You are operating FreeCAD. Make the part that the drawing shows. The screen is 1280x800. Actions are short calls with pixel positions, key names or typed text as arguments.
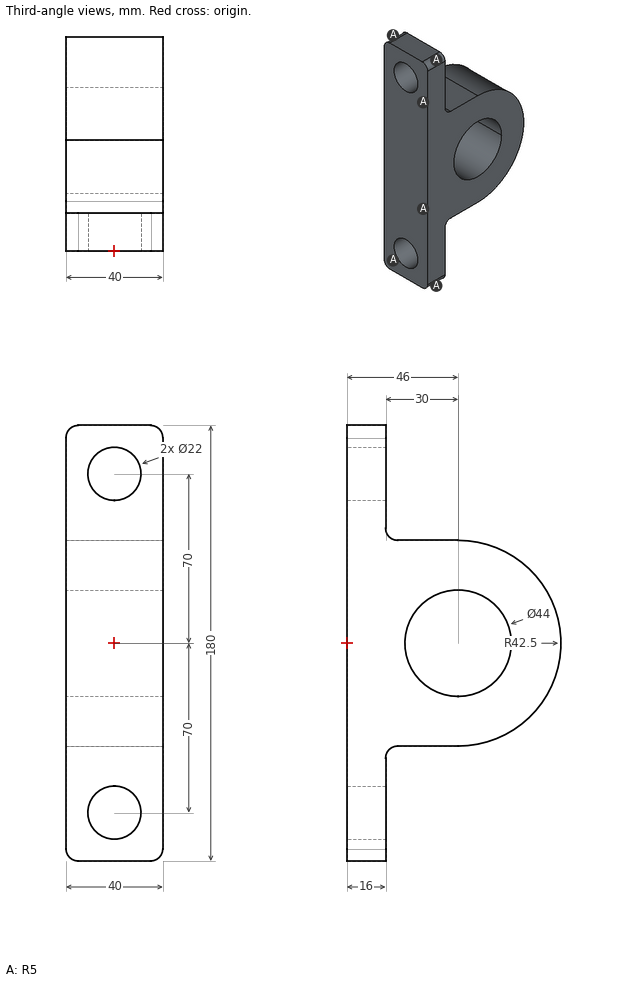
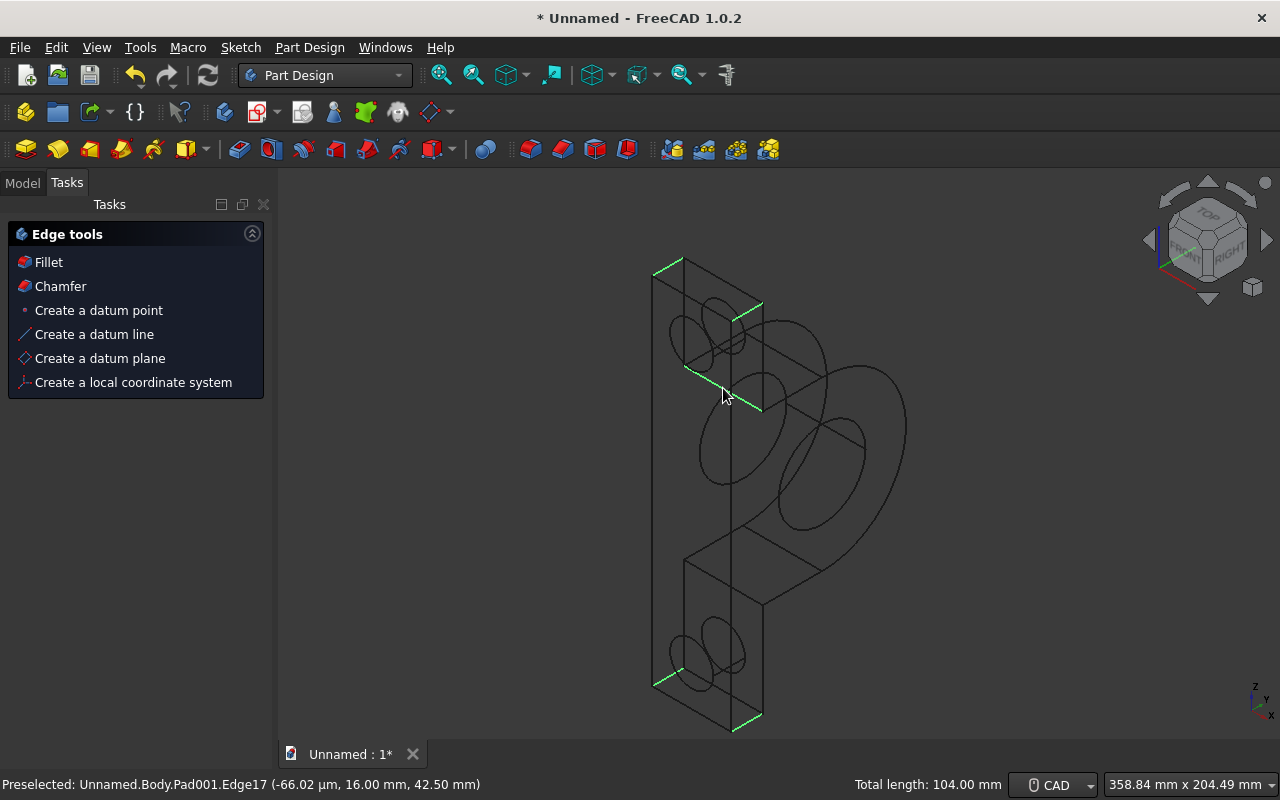
click(723, 582, ctrl)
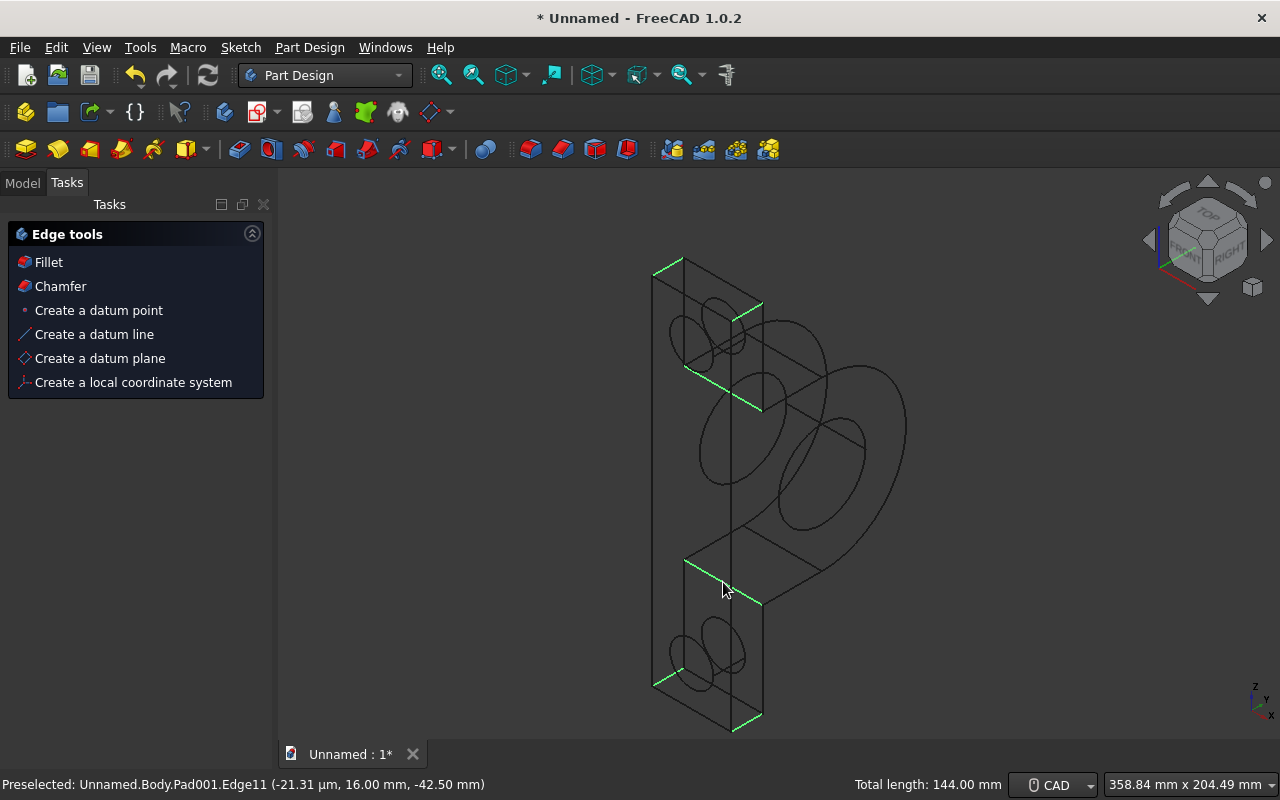
key(v)
key(1)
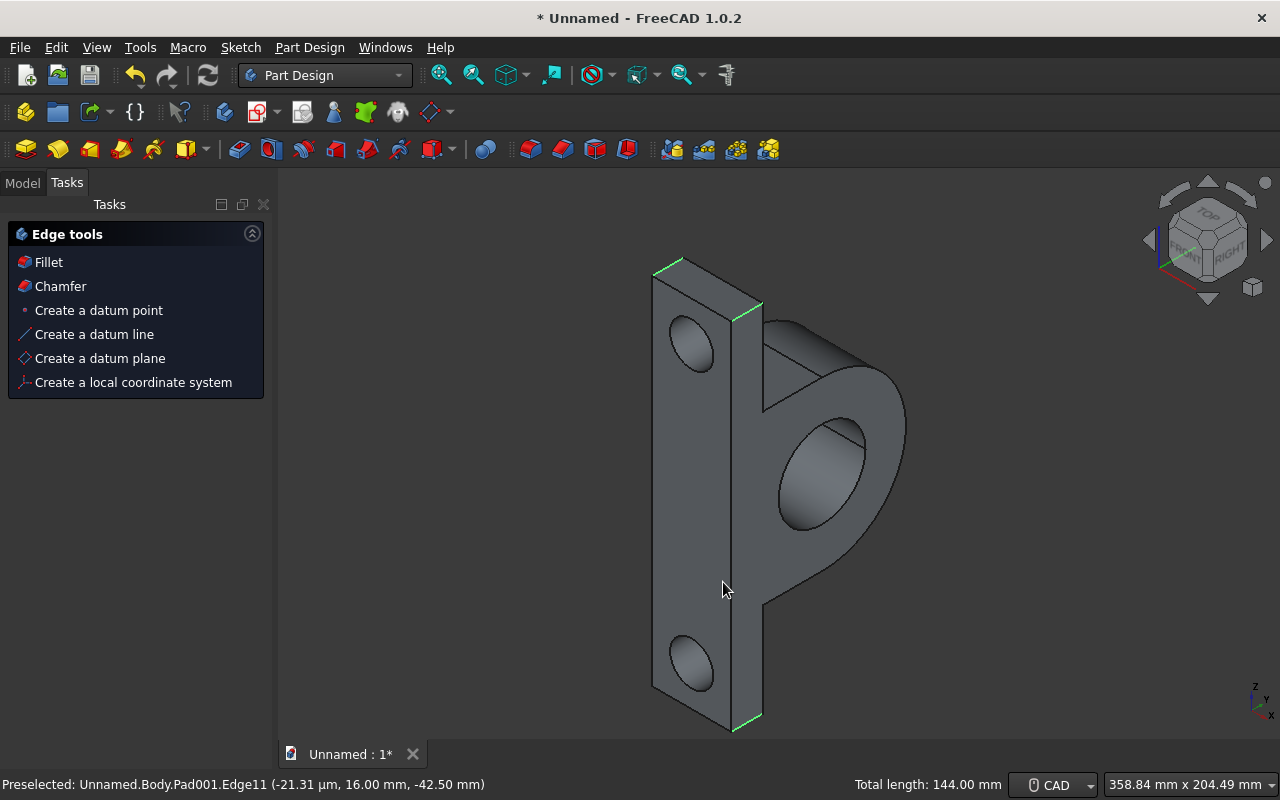
click(532, 150)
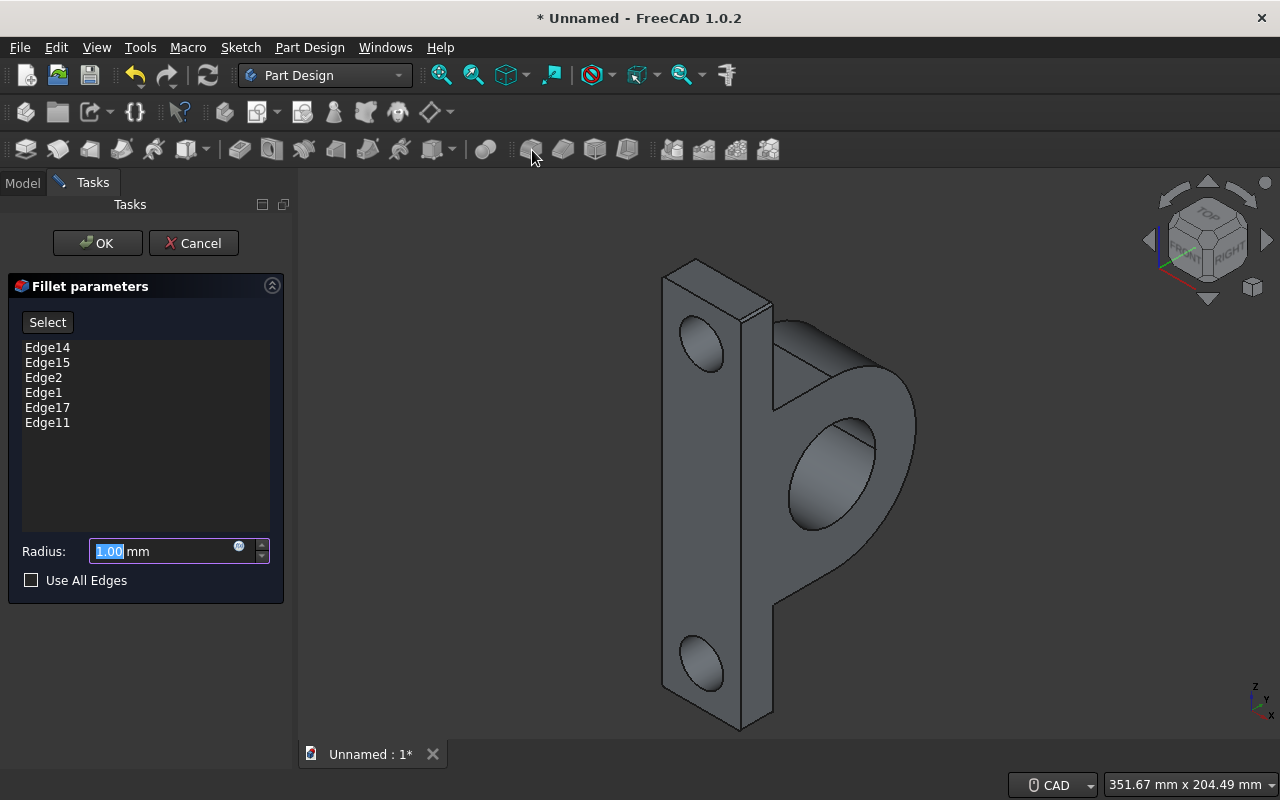
text(5)
key(Tab)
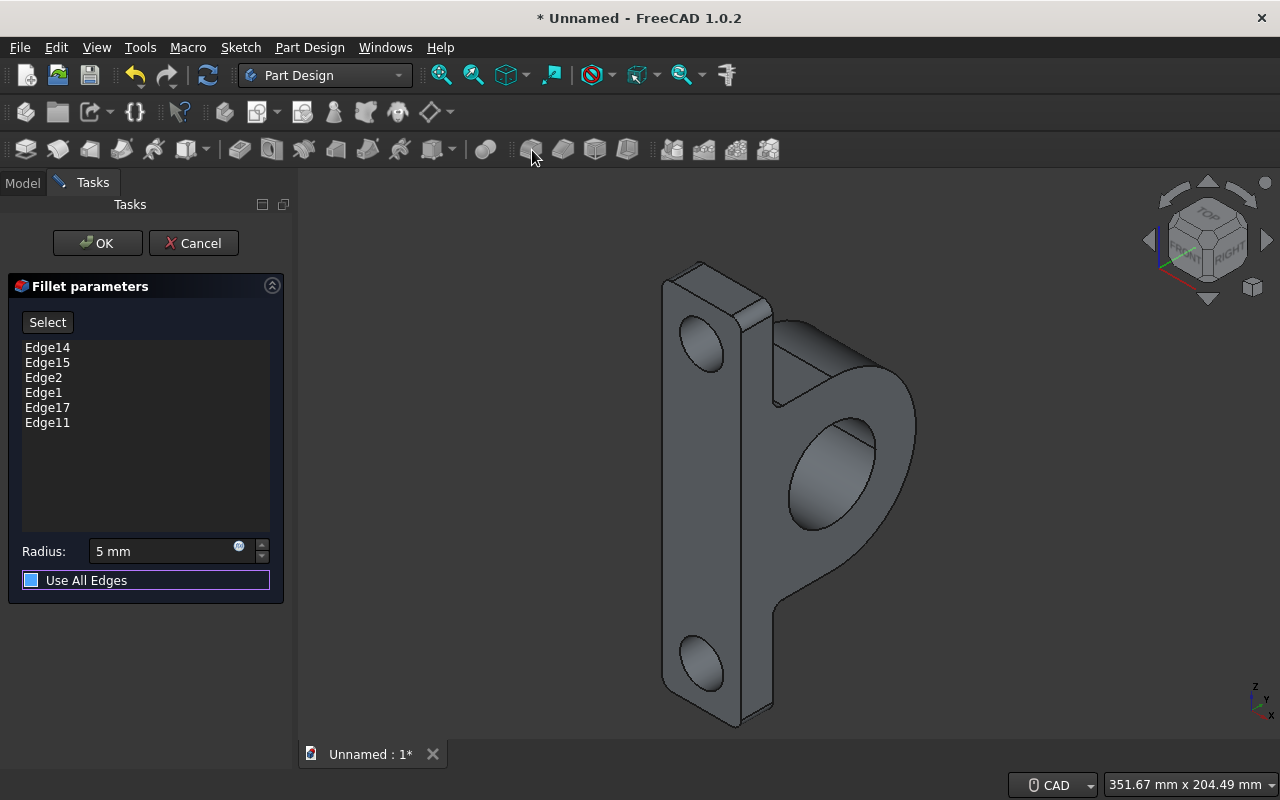
click(98, 243)